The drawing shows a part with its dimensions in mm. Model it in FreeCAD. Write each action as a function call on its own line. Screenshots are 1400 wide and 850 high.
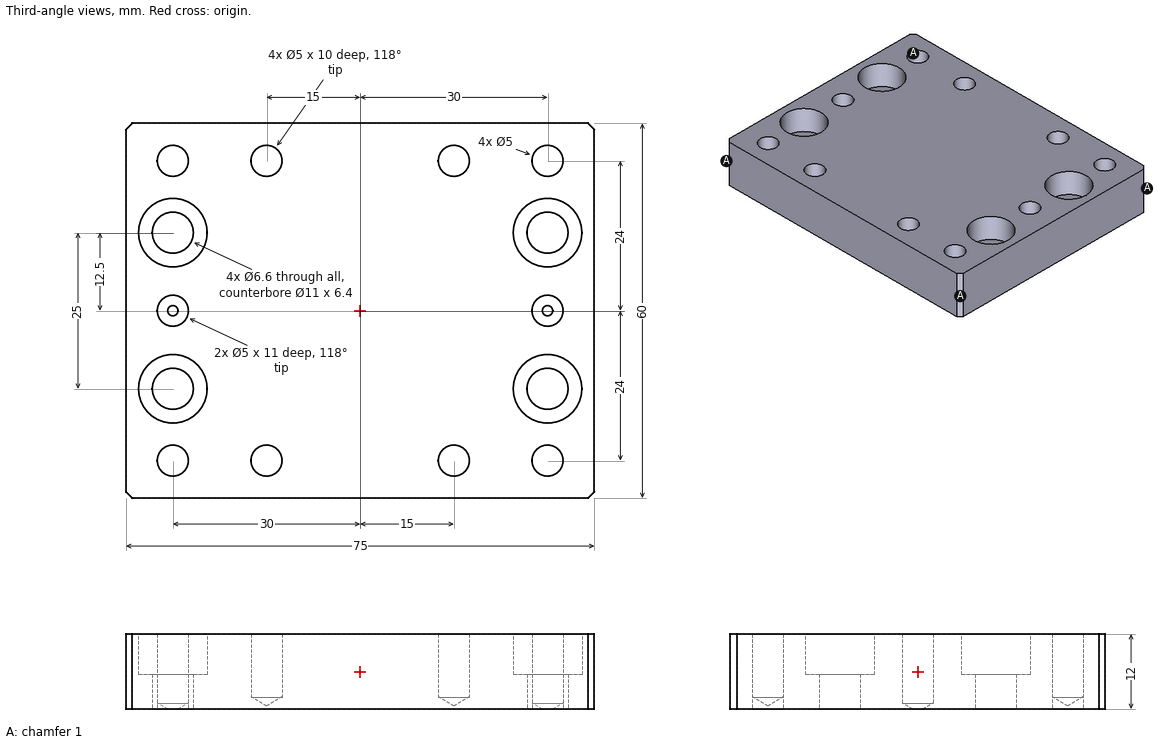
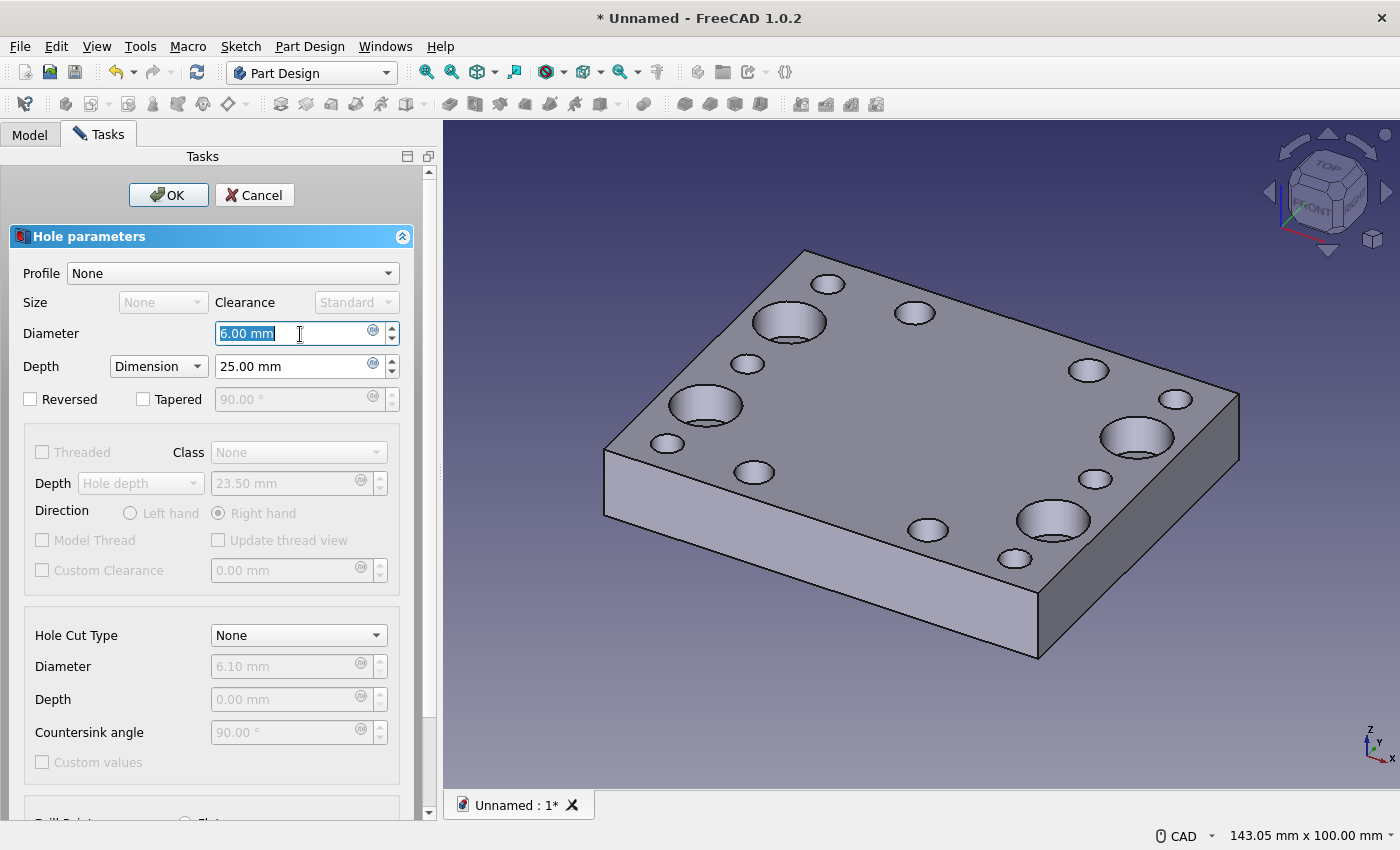
text(5)
key(Tab)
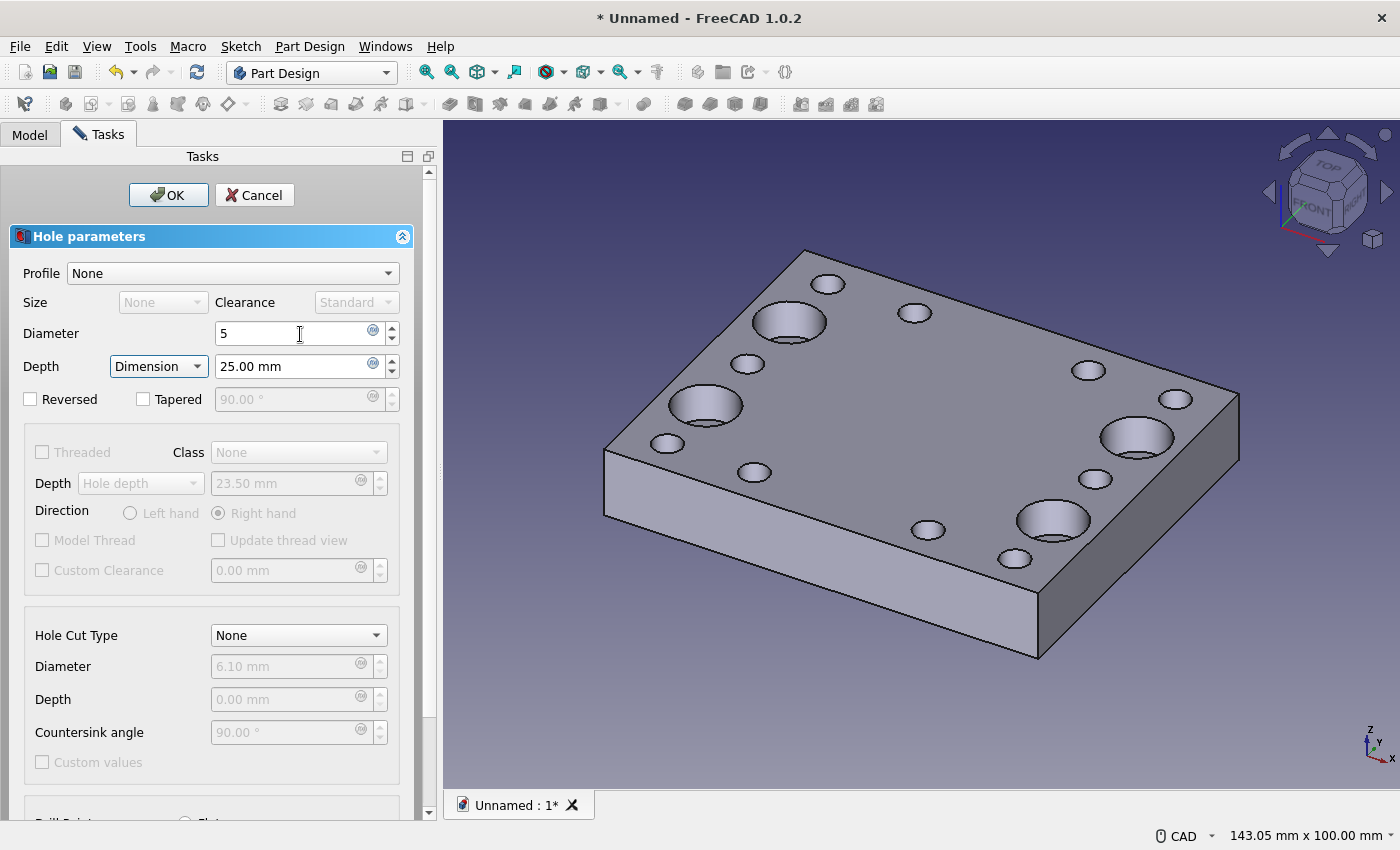
triple_click(300, 366)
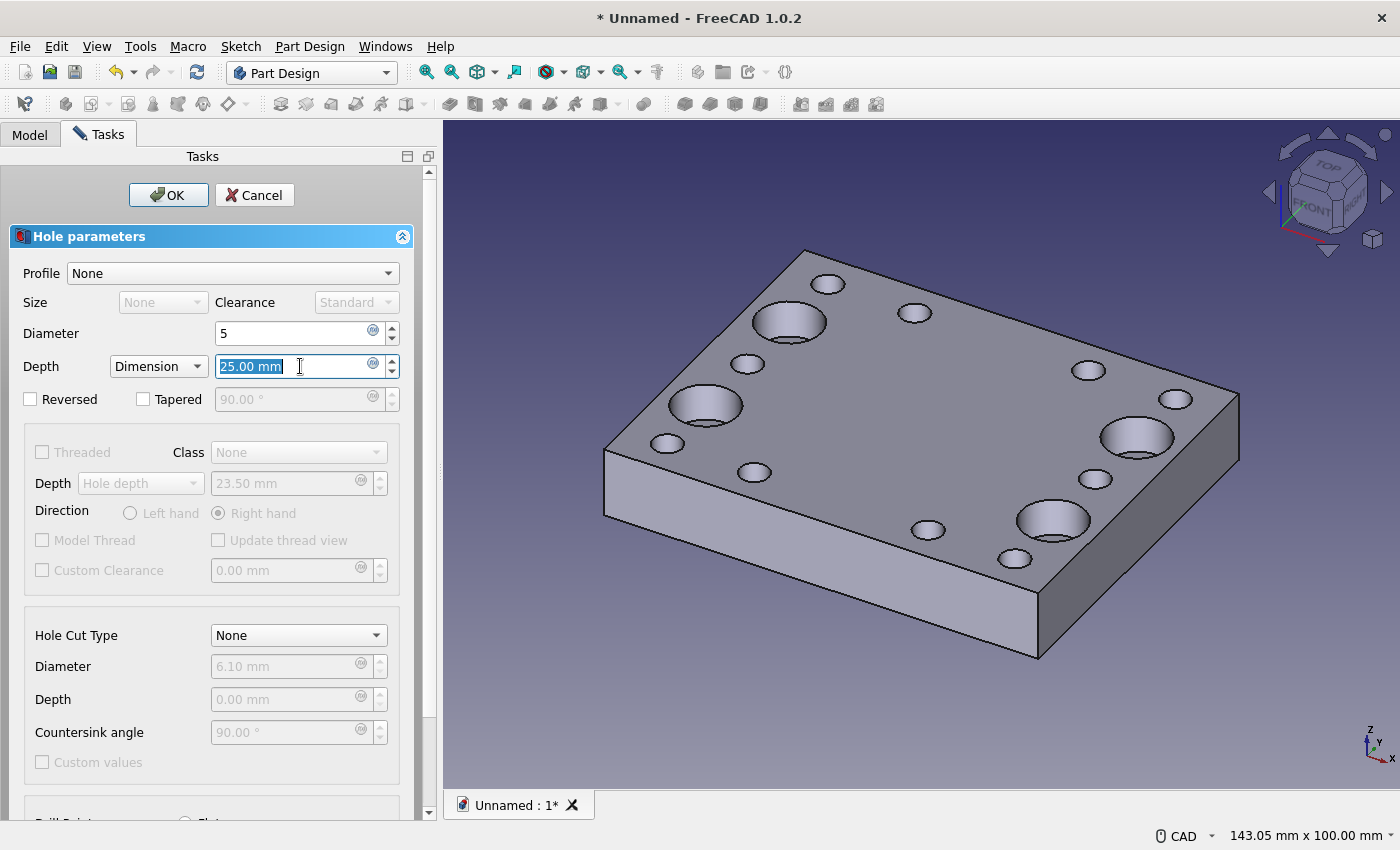
text(10)
key(Tab)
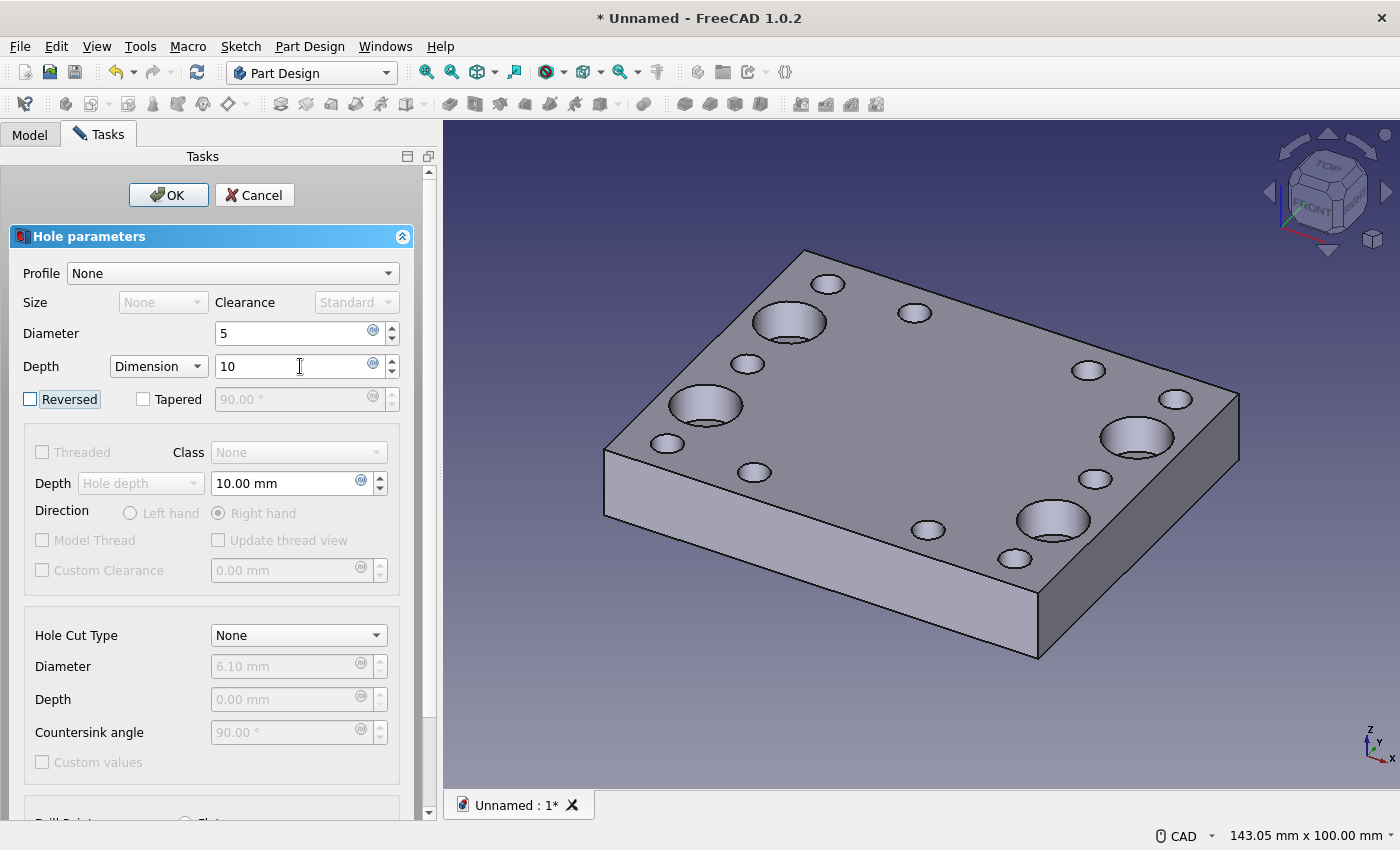
click(169, 195)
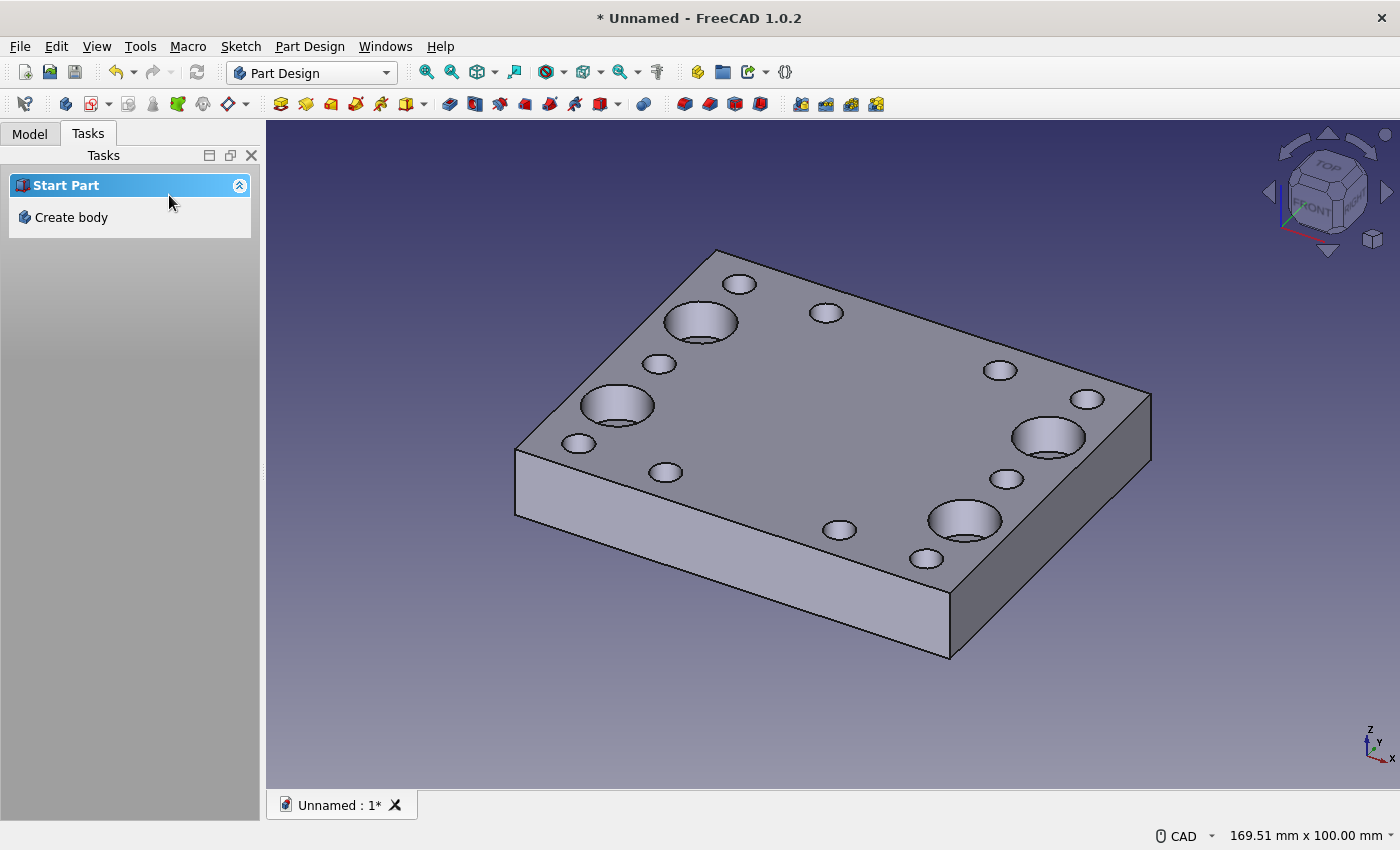
click(950, 625)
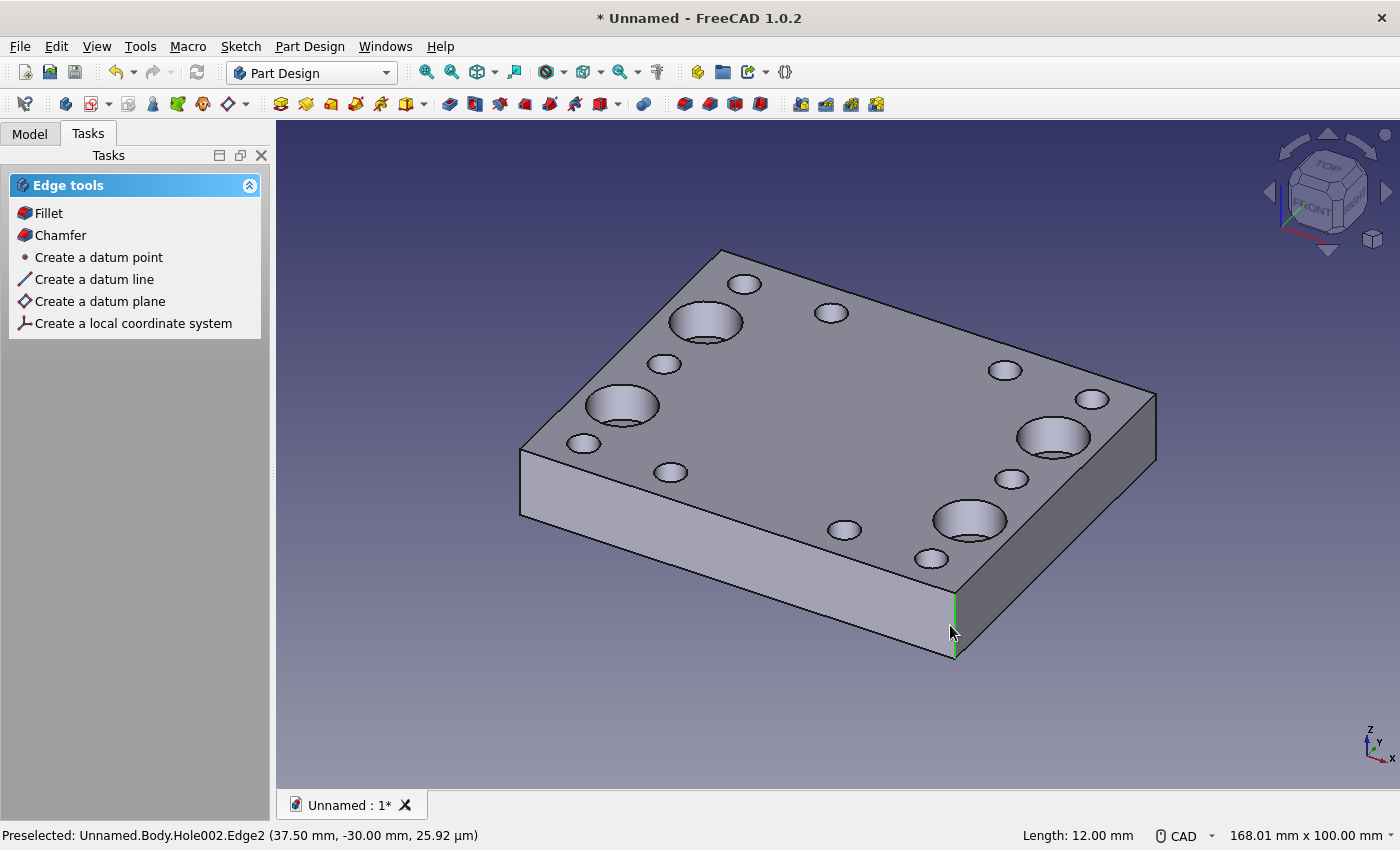
key(0)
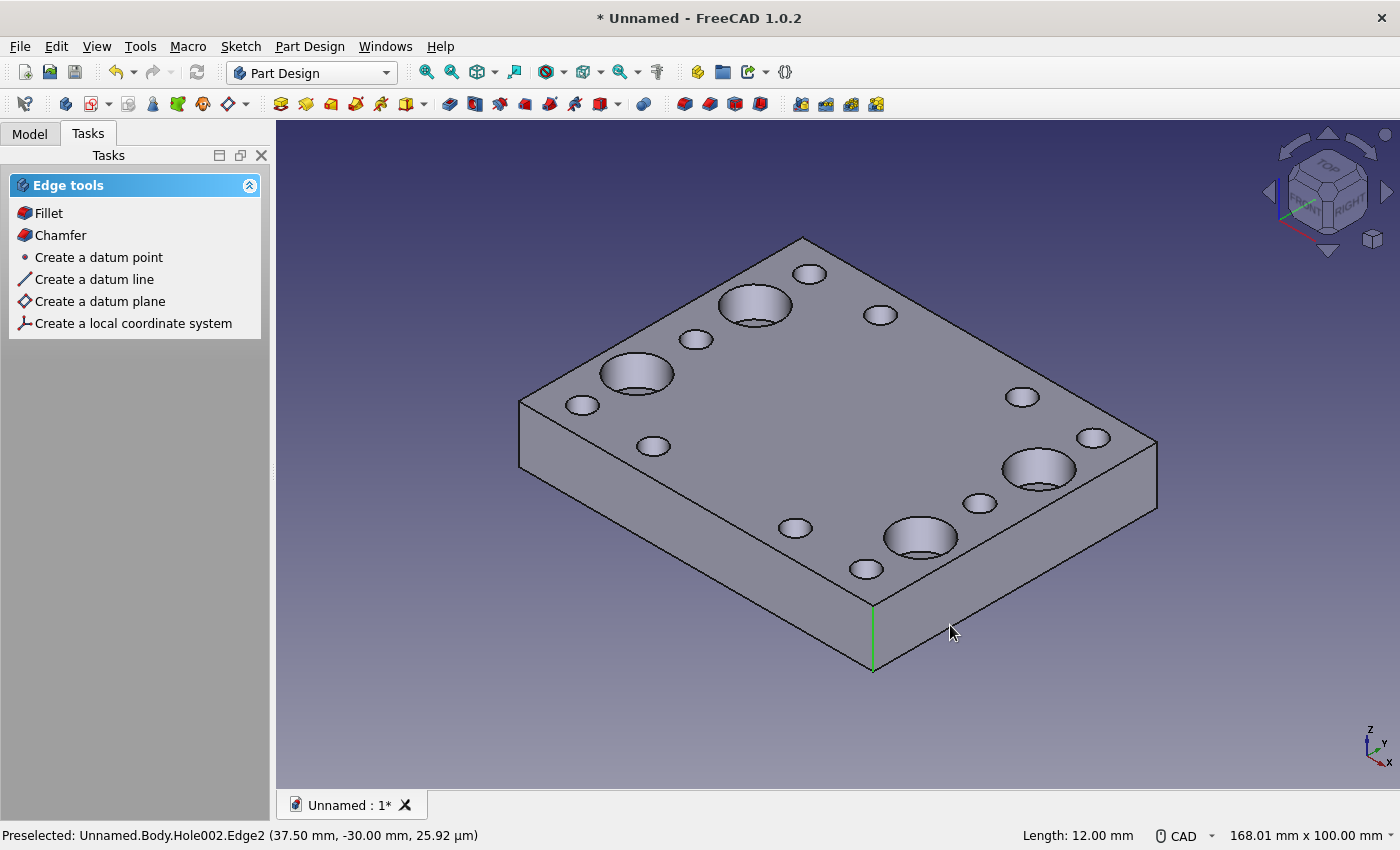
key(2)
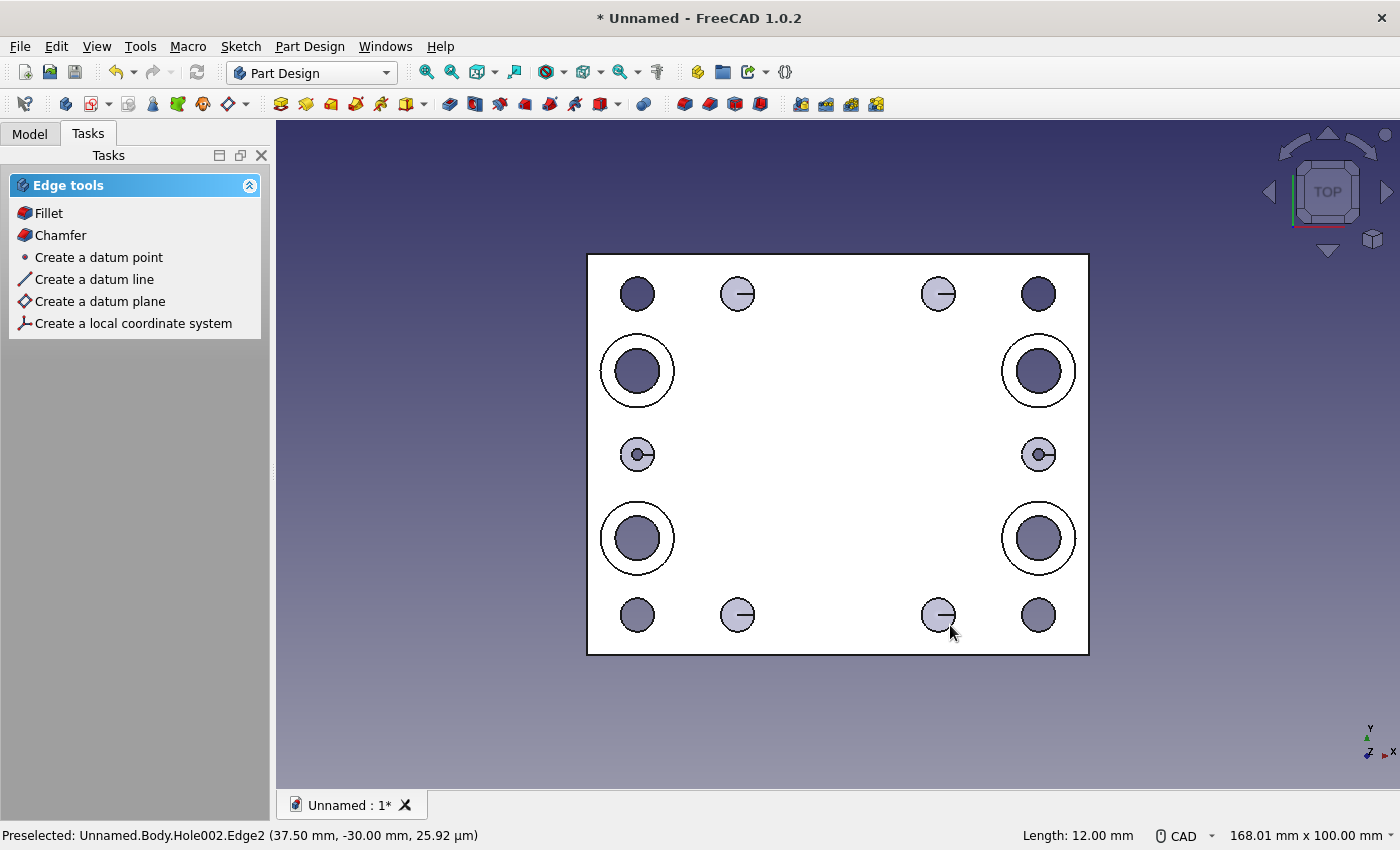
key(1)